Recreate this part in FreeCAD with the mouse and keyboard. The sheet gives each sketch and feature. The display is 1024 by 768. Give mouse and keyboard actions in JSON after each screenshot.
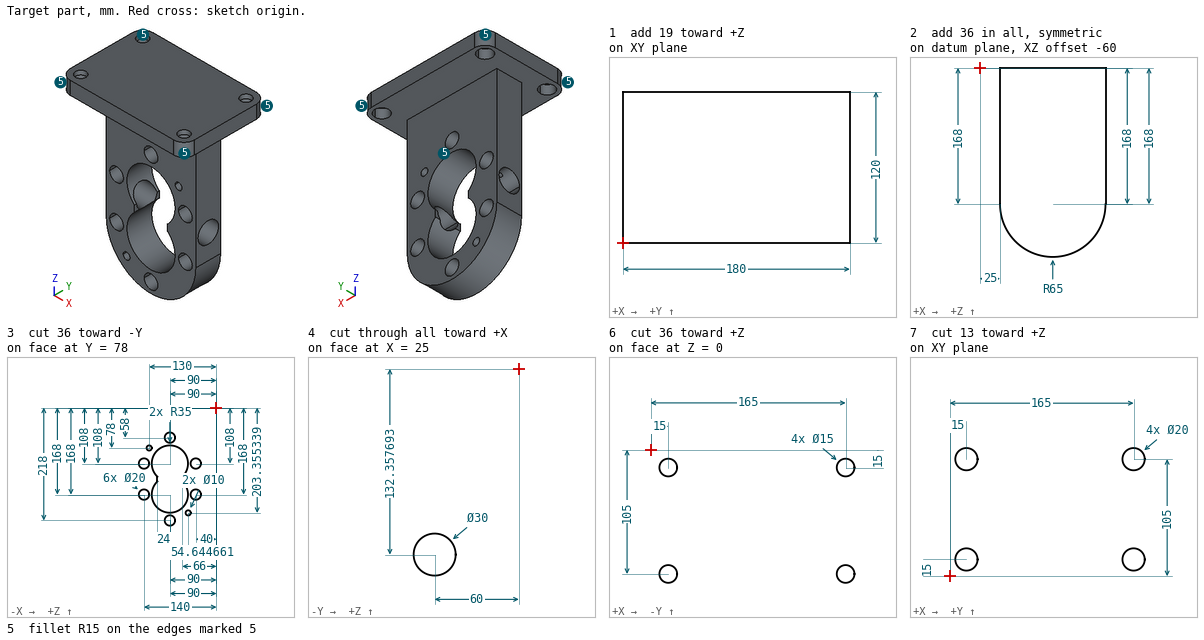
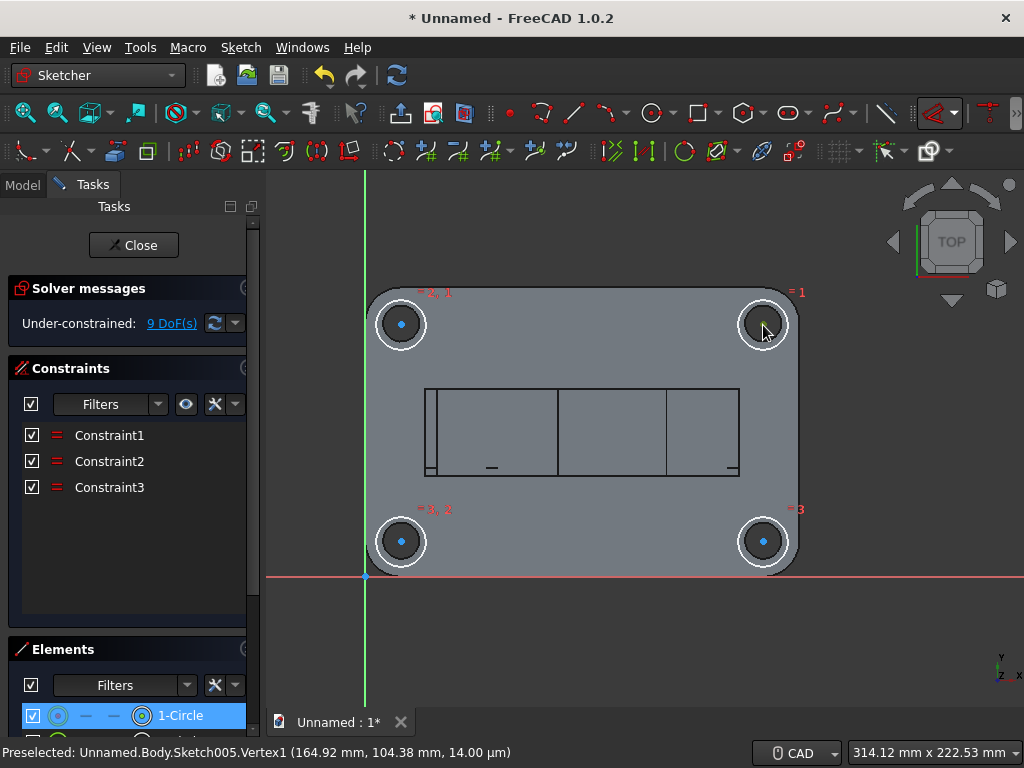
{"action": "left_click", "coordinate": [401, 325]}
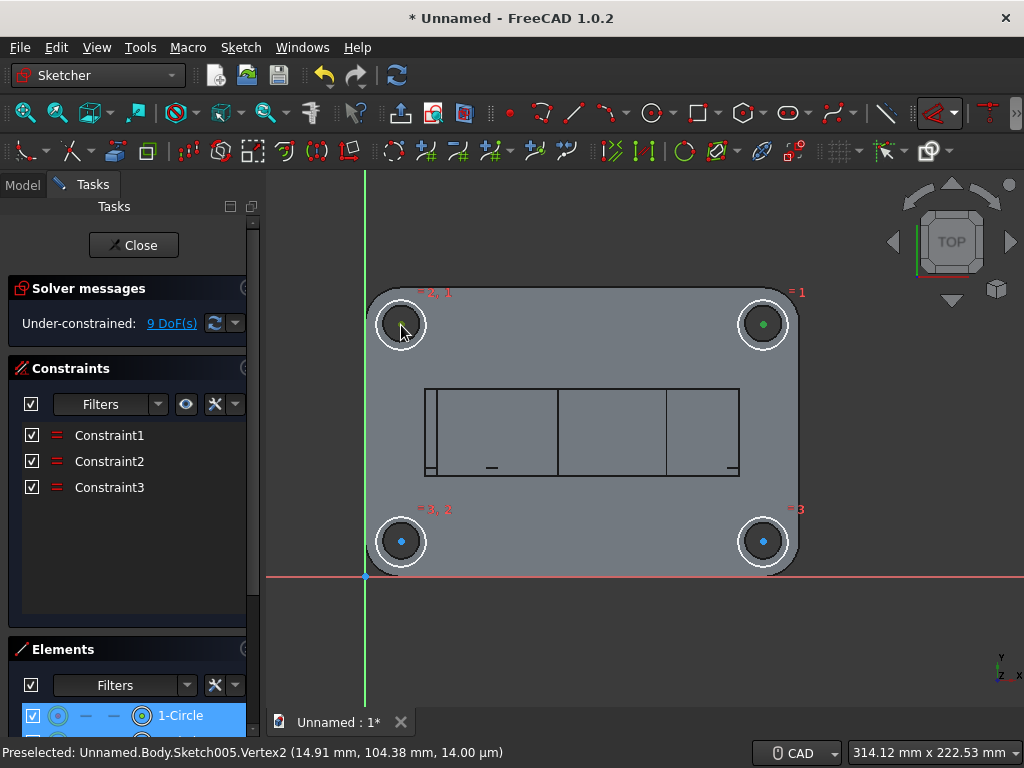
{"action": "key", "text": "h"}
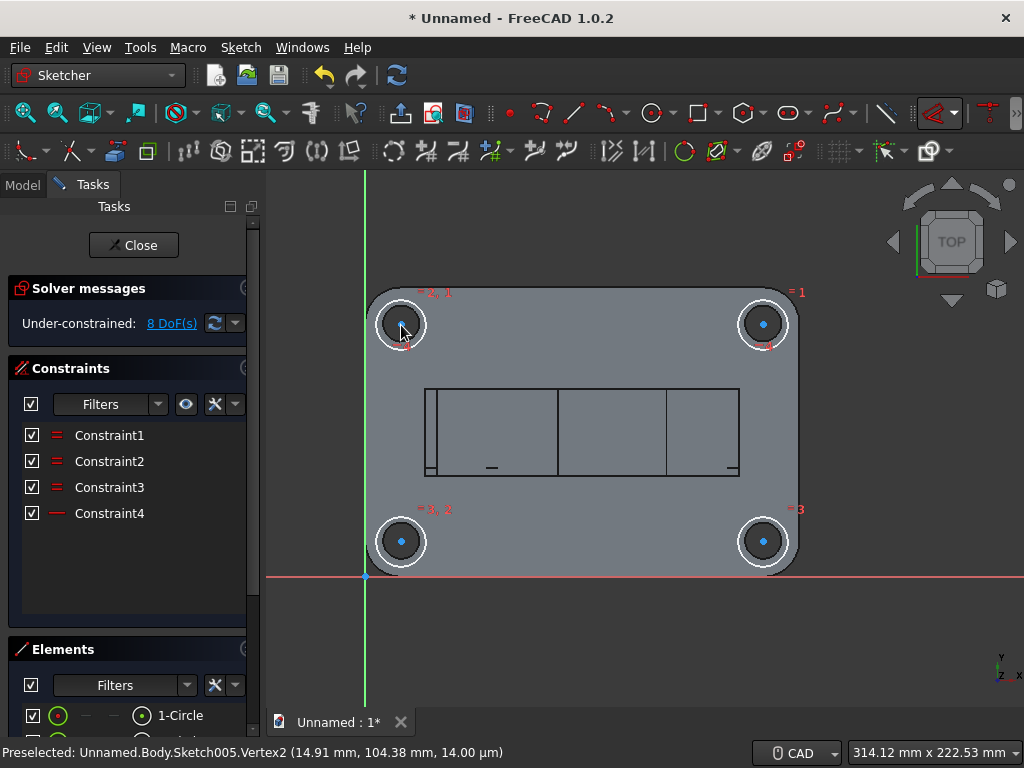
{"action": "left_click", "coordinate": [401, 325]}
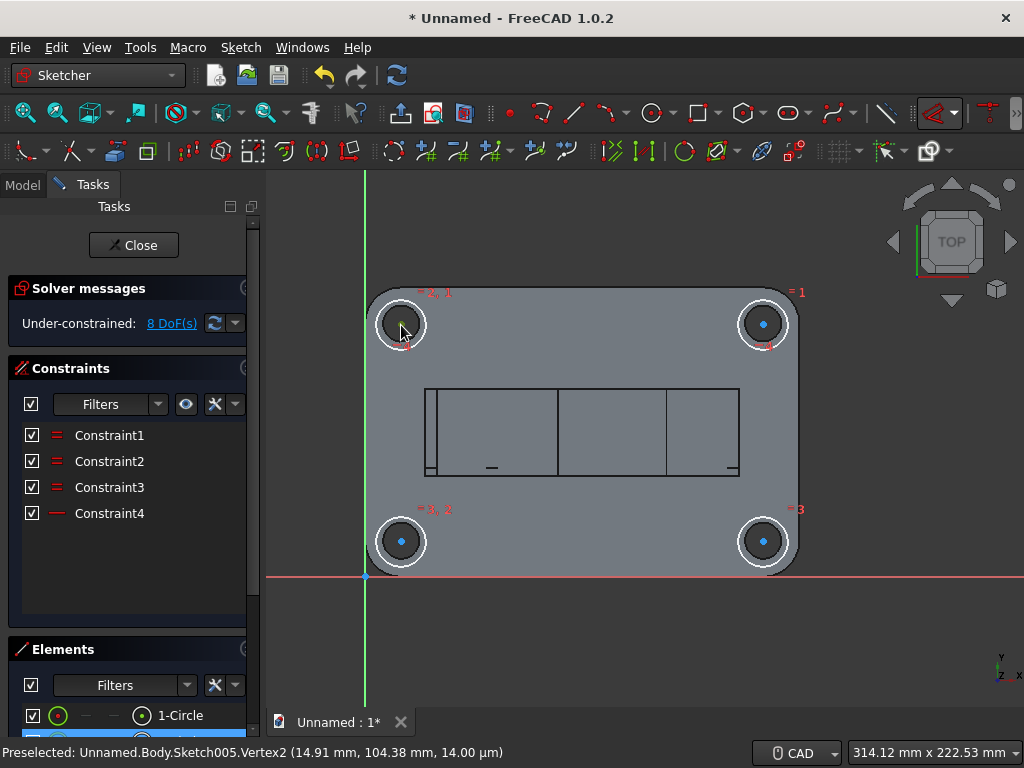
{"action": "left_click", "coordinate": [401, 542]}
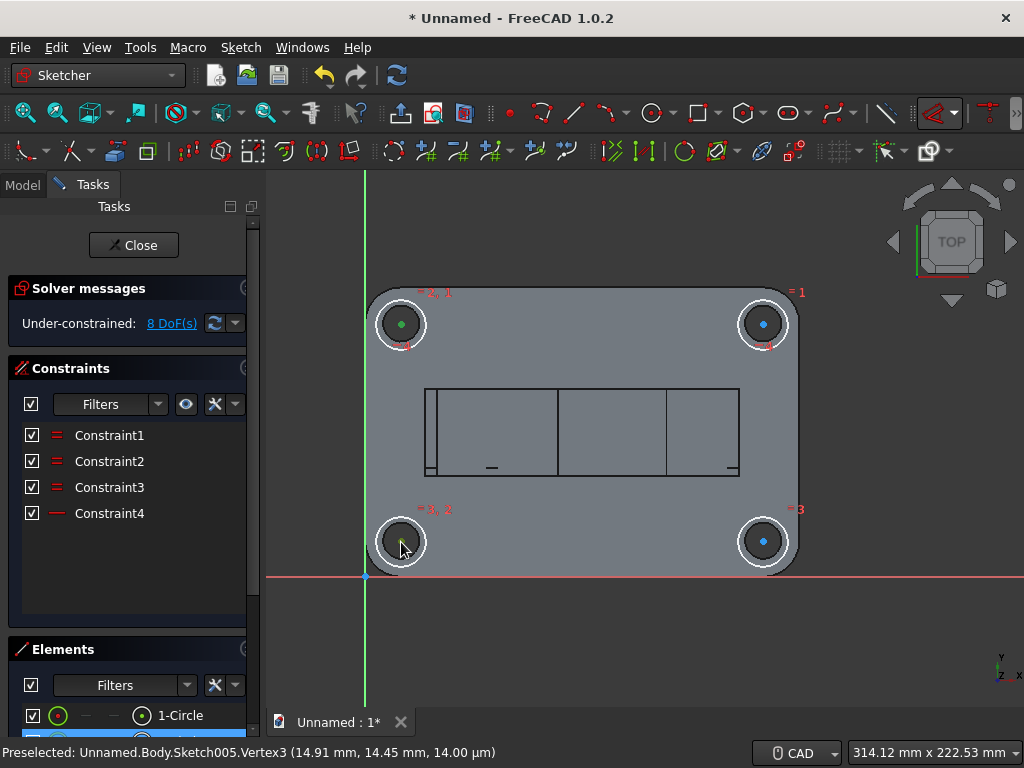
{"action": "key", "text": "v"}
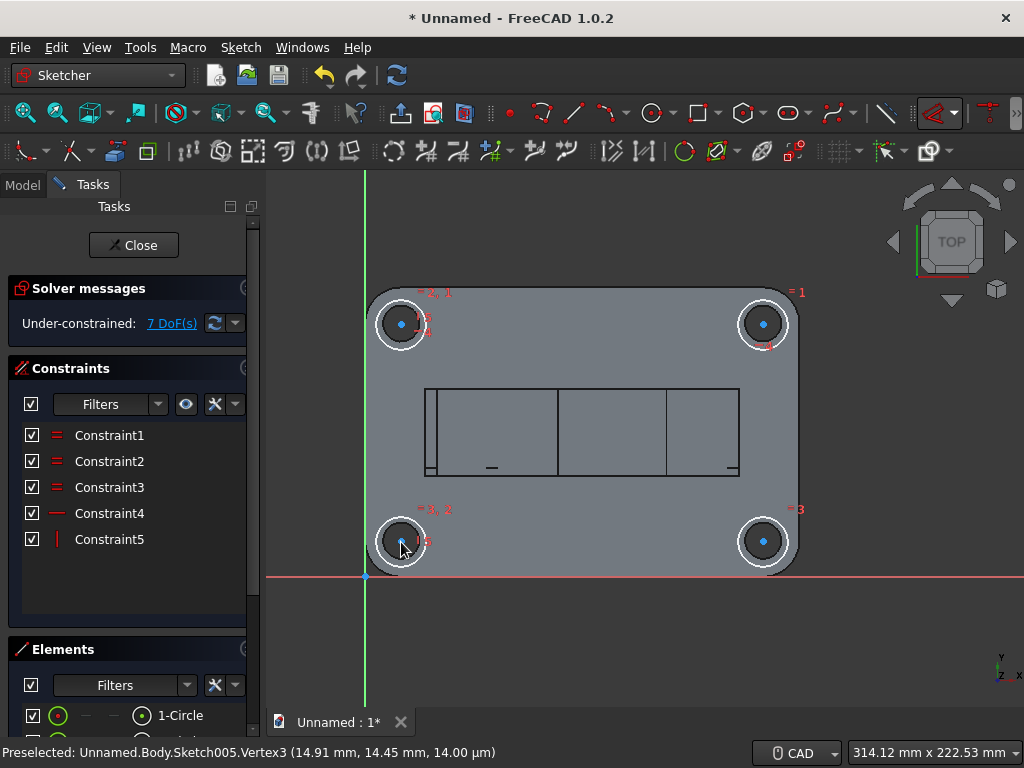
{"action": "left_click", "coordinate": [763, 325]}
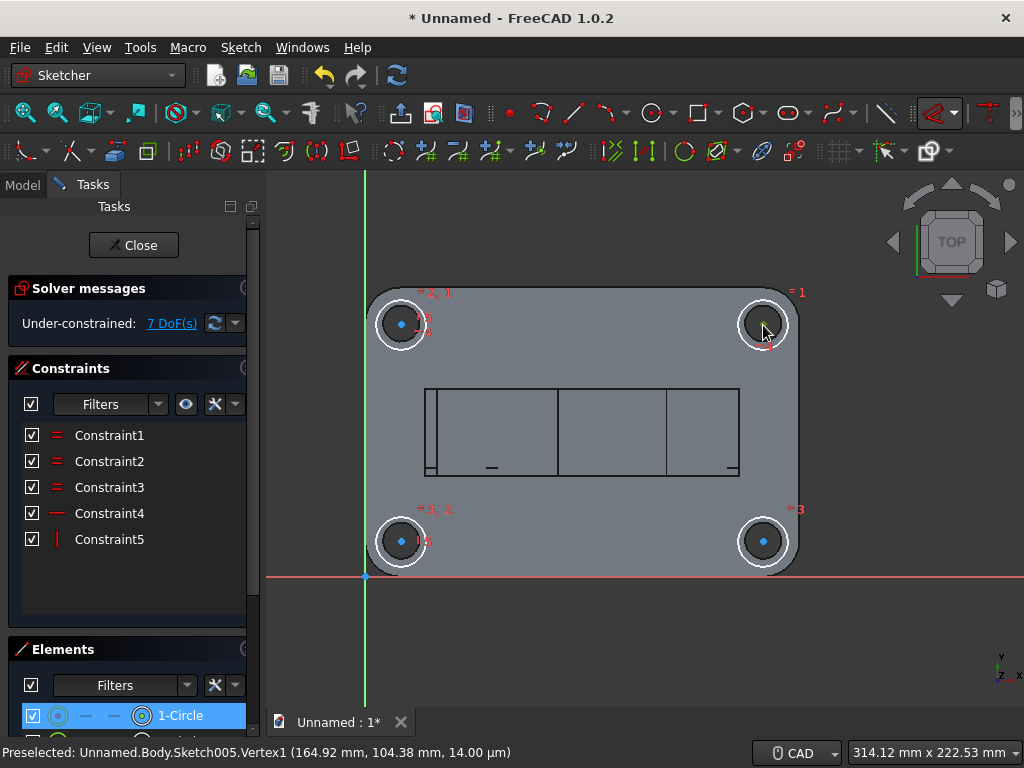
{"action": "left_click", "coordinate": [763, 542]}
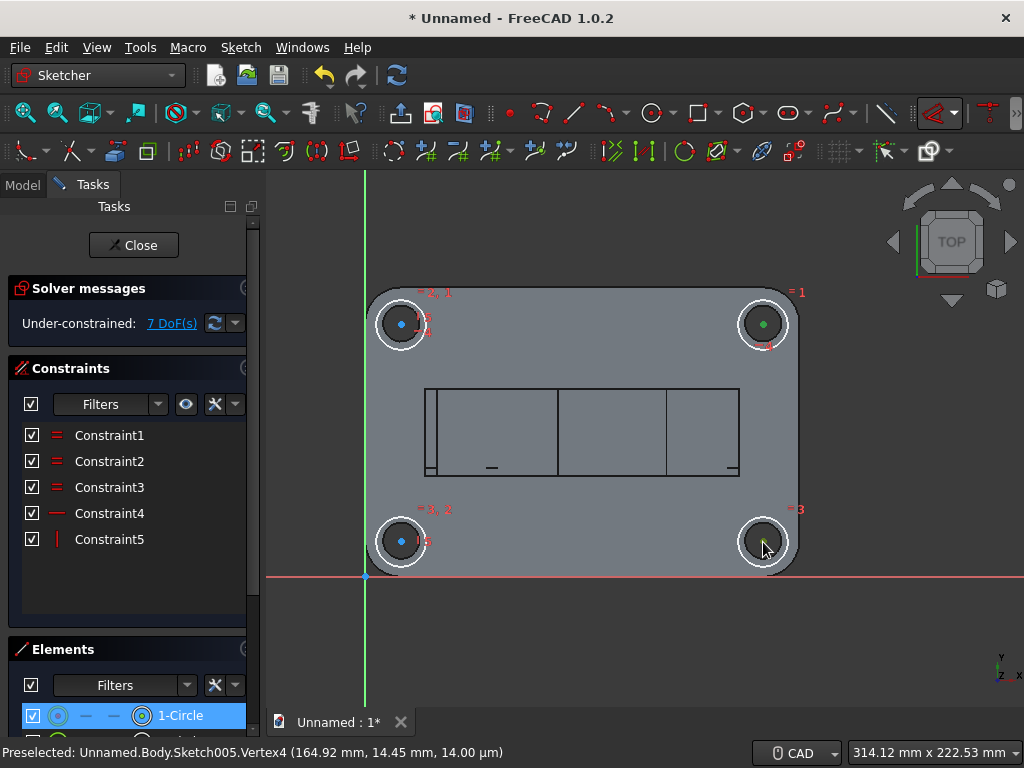
{"action": "key", "text": "v"}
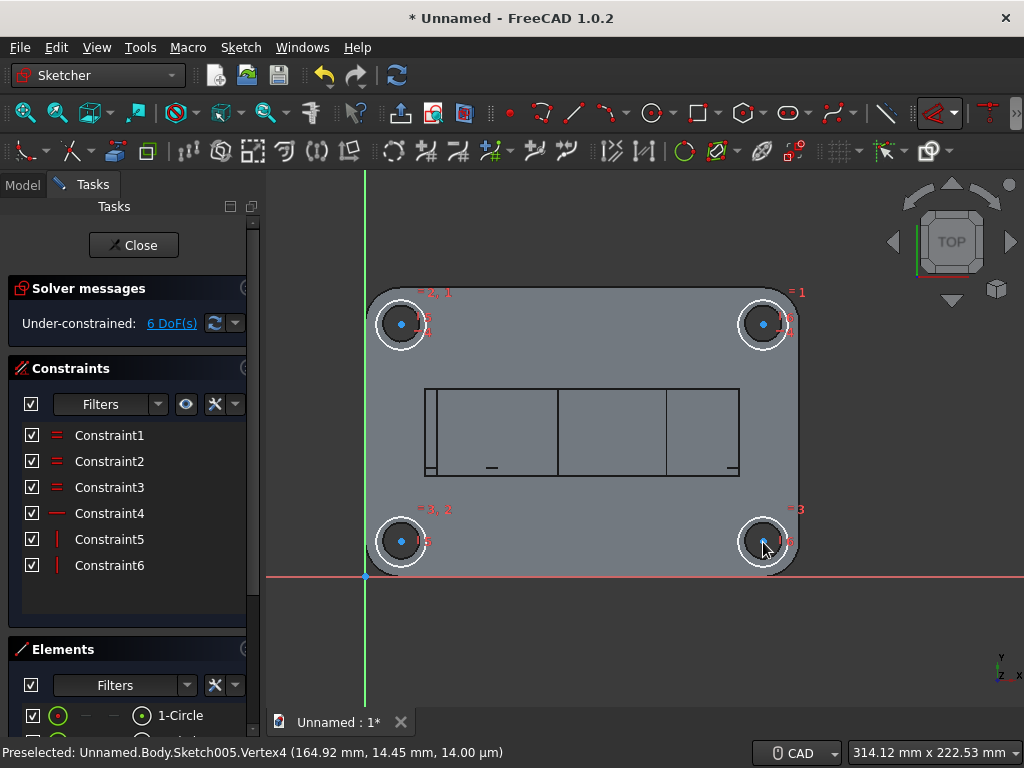
{"action": "left_click", "coordinate": [401, 542]}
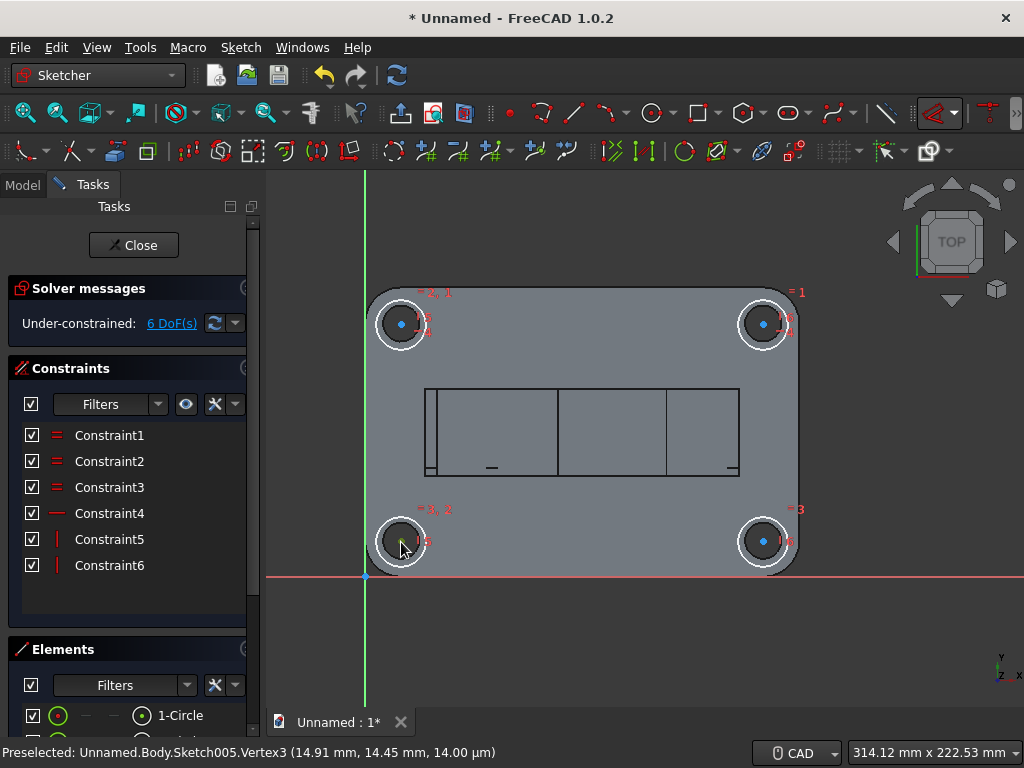
{"action": "left_click", "coordinate": [763, 542]}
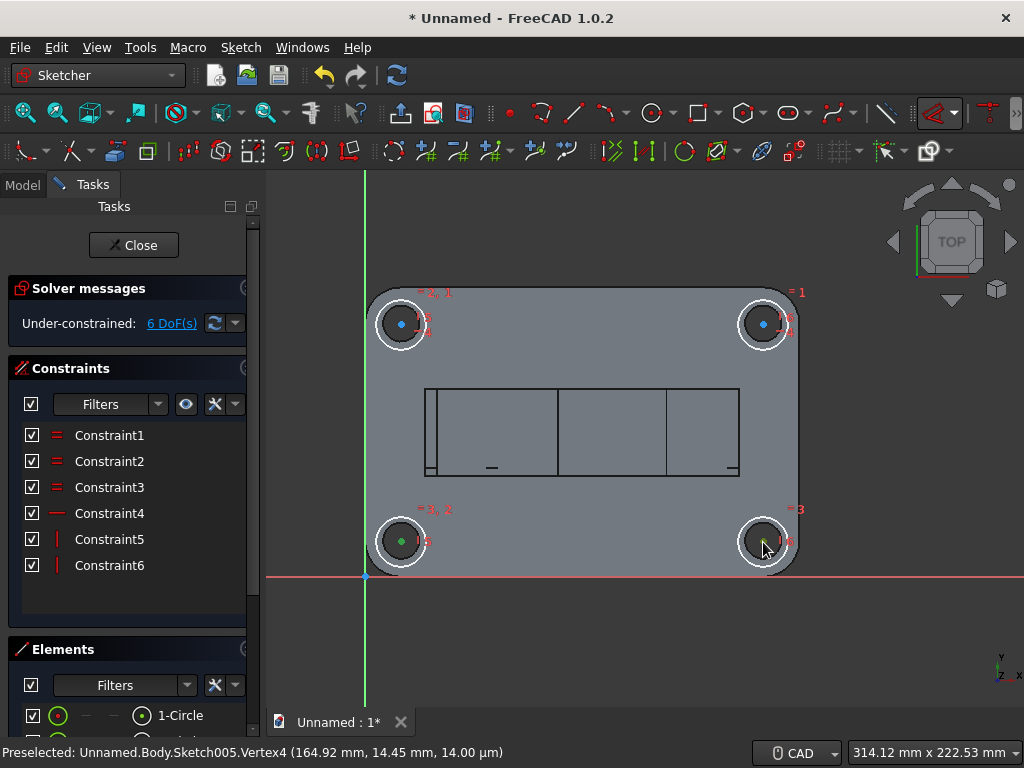
{"action": "key", "text": "h"}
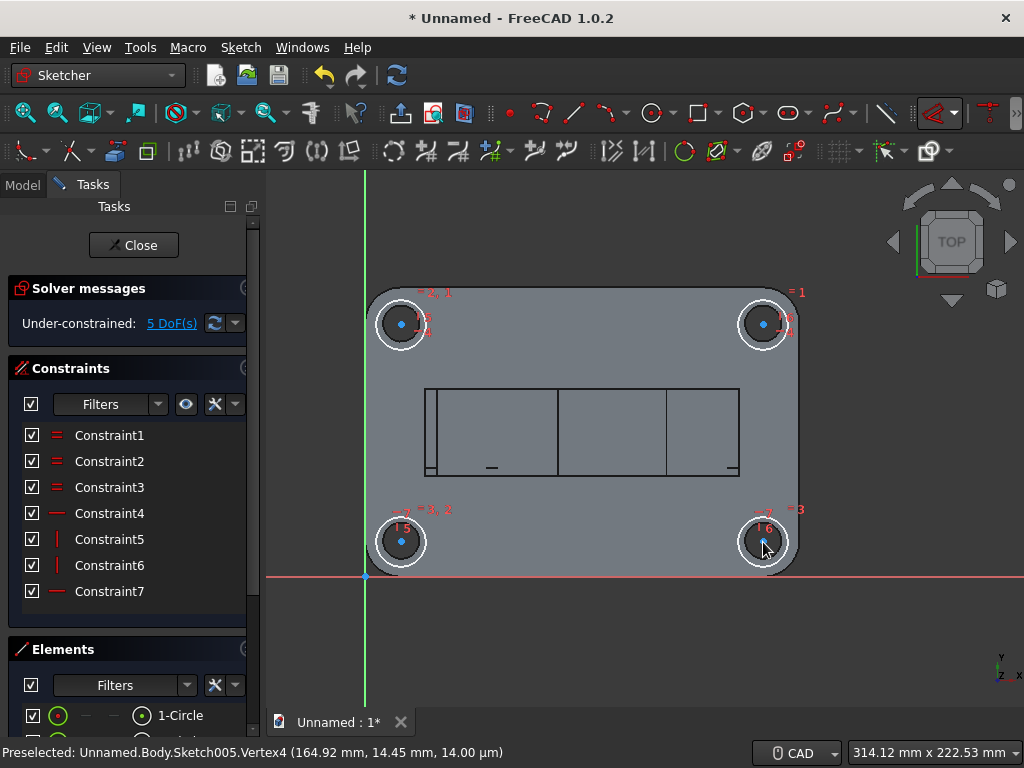
{"action": "left_click", "coordinate": [780, 307]}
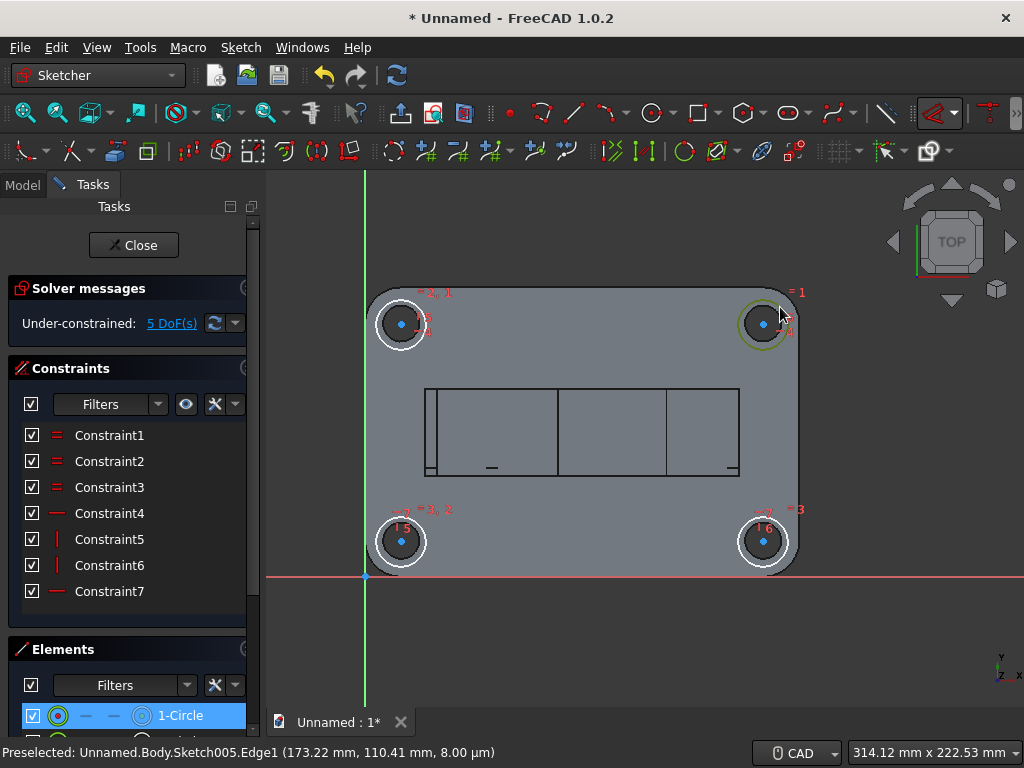
{"action": "key", "text": "k o"}